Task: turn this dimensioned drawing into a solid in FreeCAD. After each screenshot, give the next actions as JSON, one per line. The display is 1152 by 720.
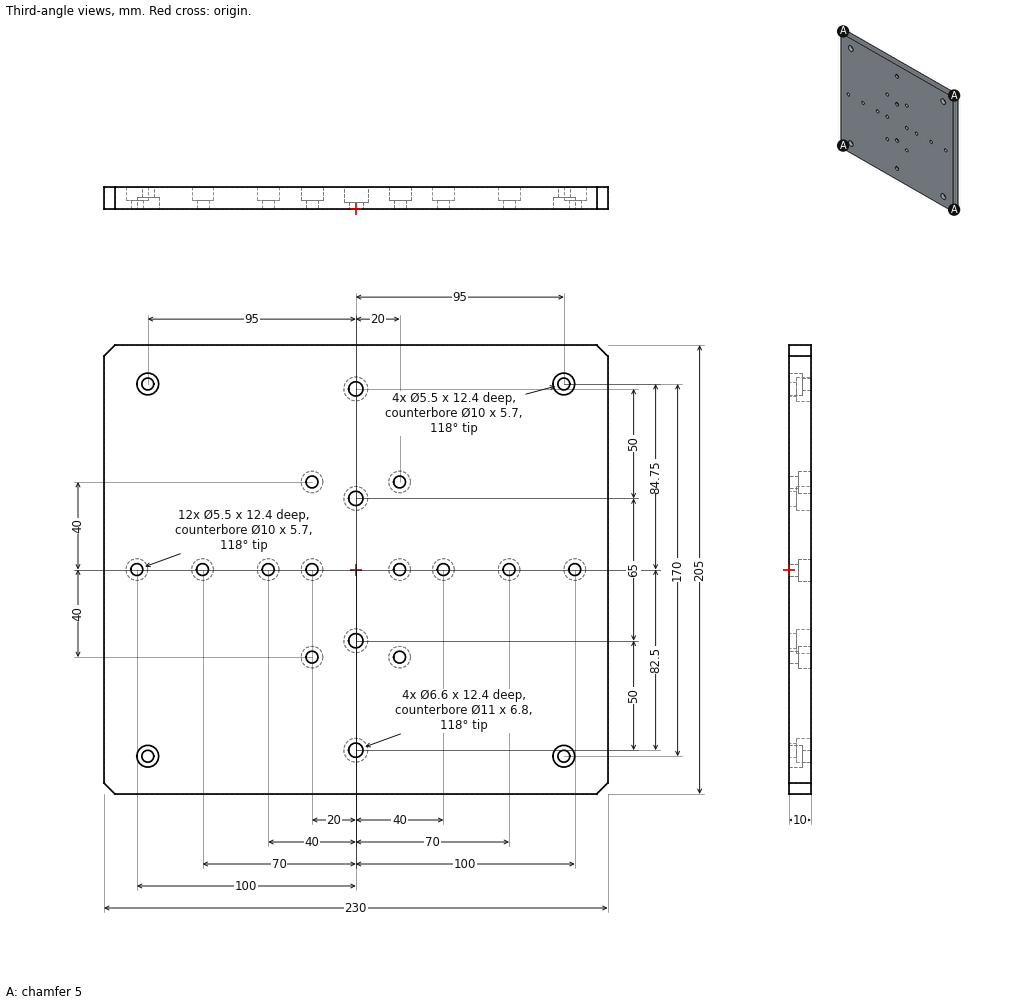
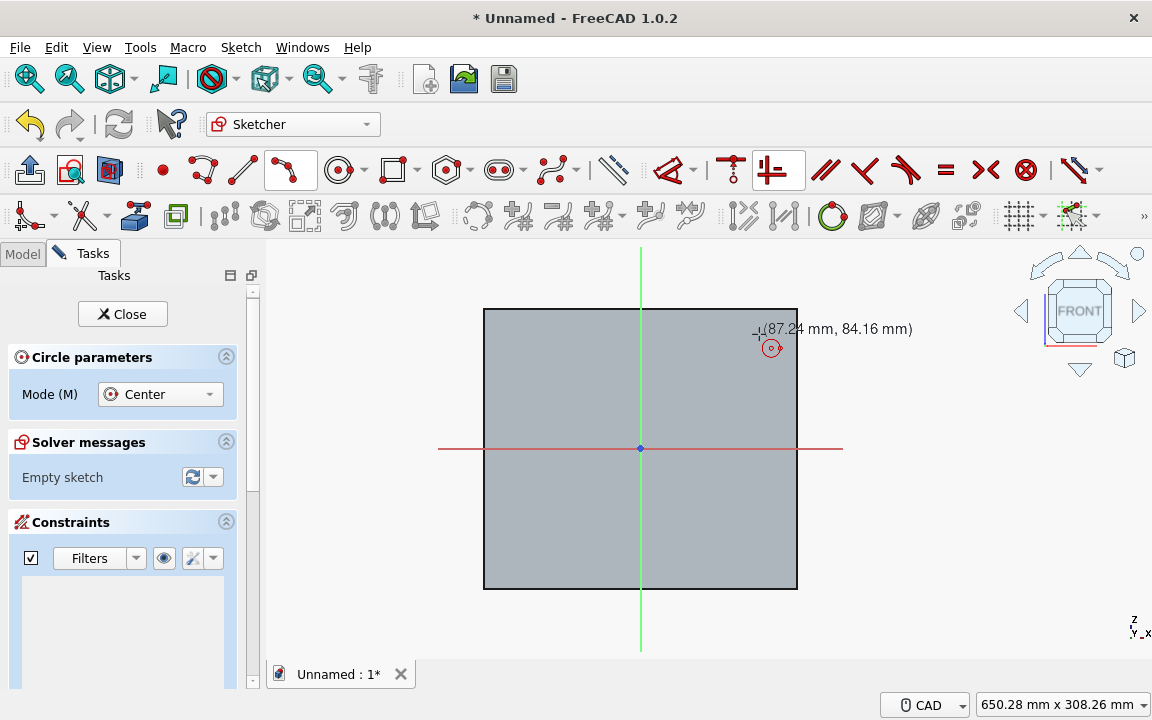
{"action": "left_click", "coordinate": [770, 334]}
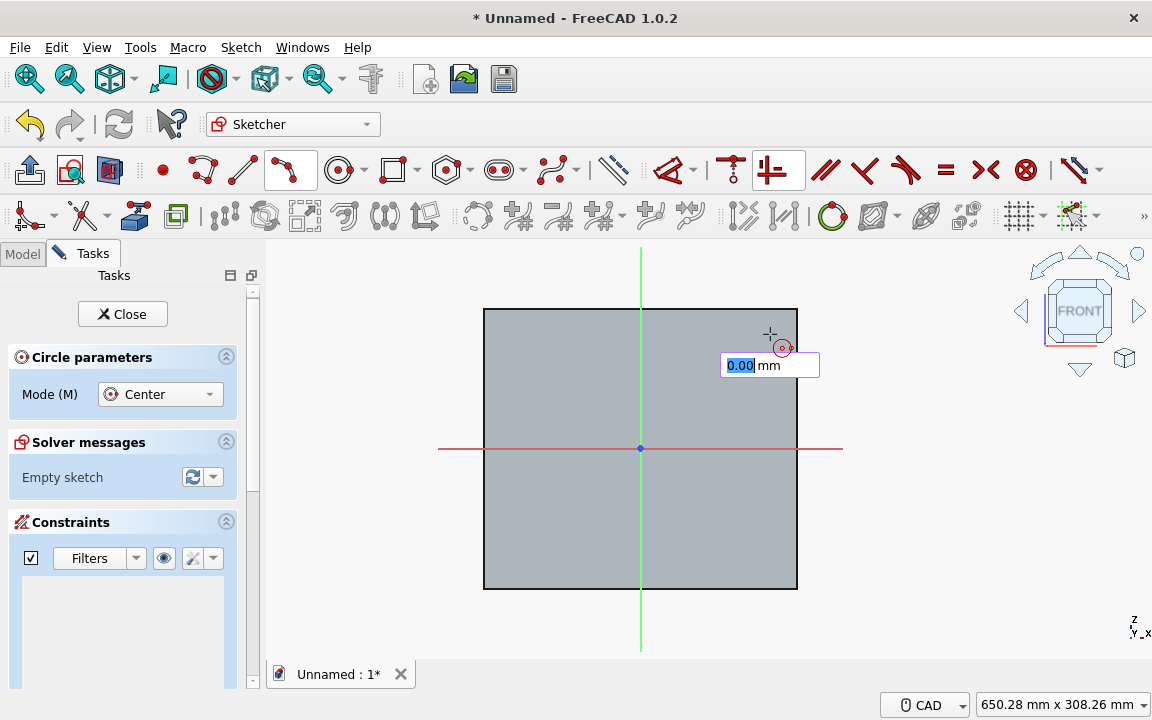
{"action": "scroll", "coordinate": [773, 331], "scroll_direction": "up", "scroll_amount": 8}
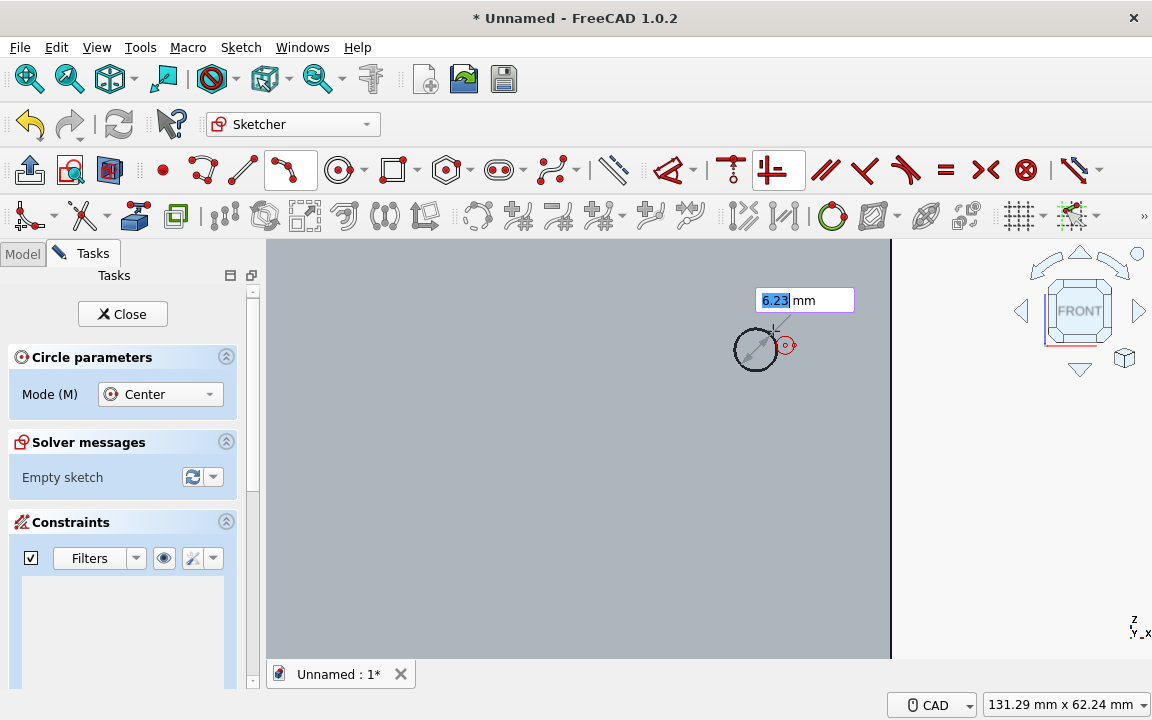
{"action": "left_click", "coordinate": [769, 330]}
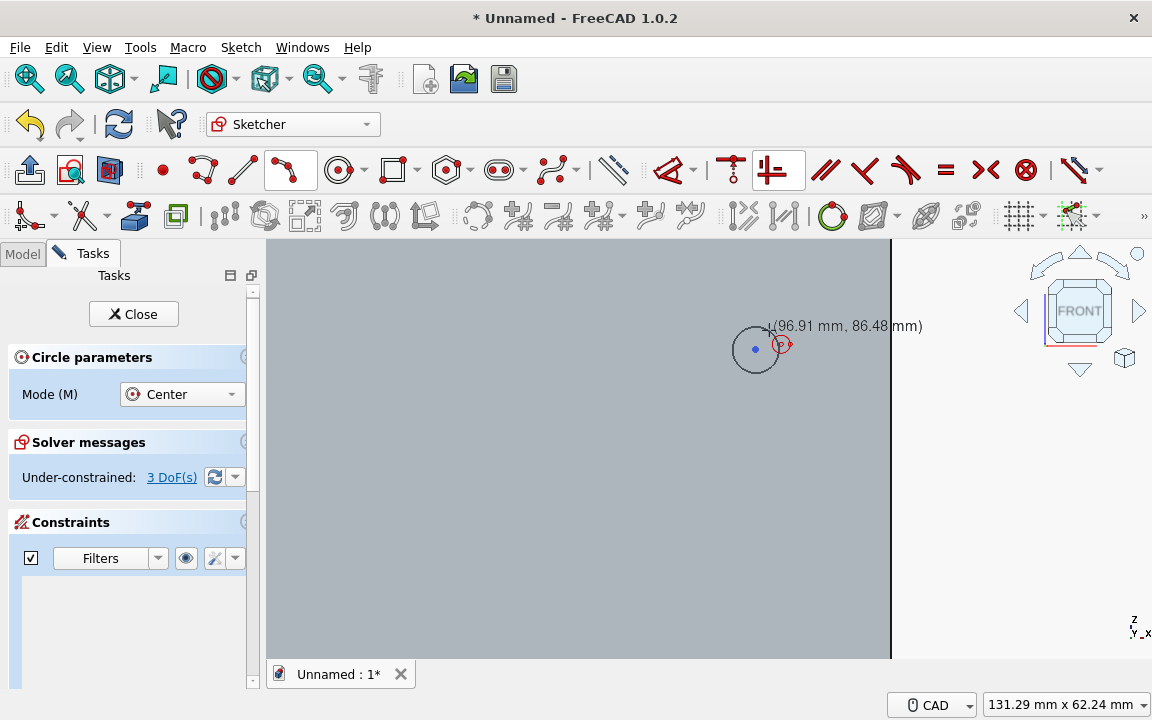
{"action": "scroll", "coordinate": [773, 331], "scroll_direction": "down", "scroll_amount": 8}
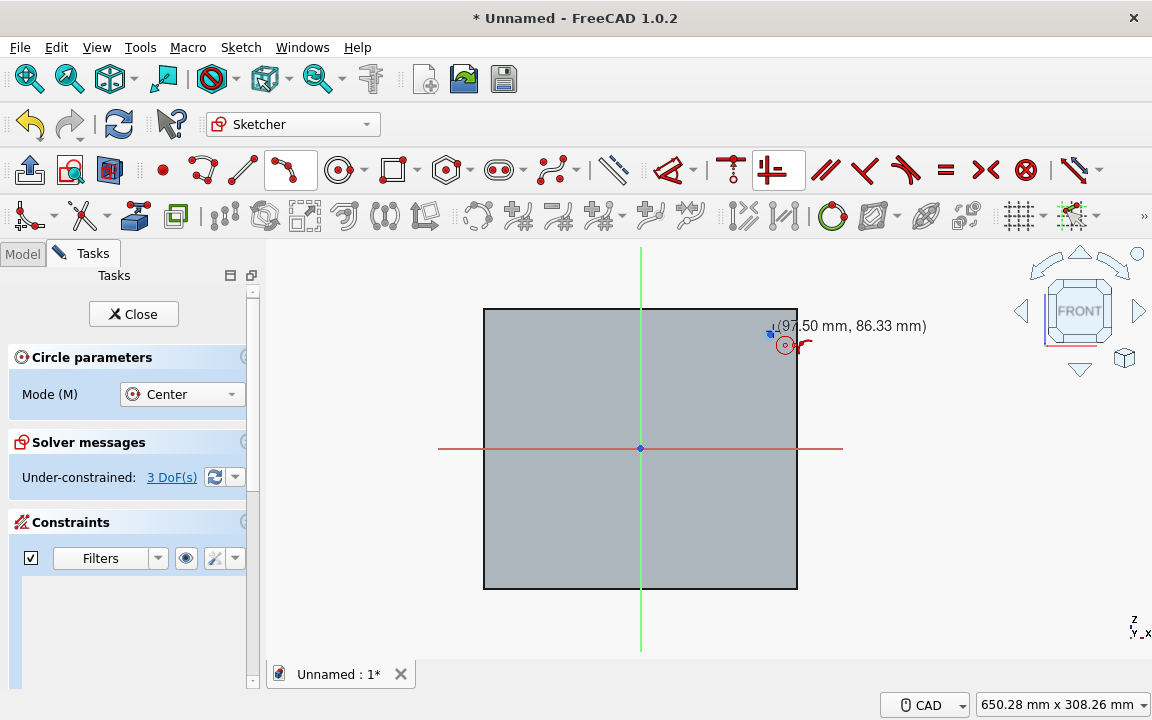
{"action": "scroll", "coordinate": [770, 565], "scroll_direction": "up", "scroll_amount": 10}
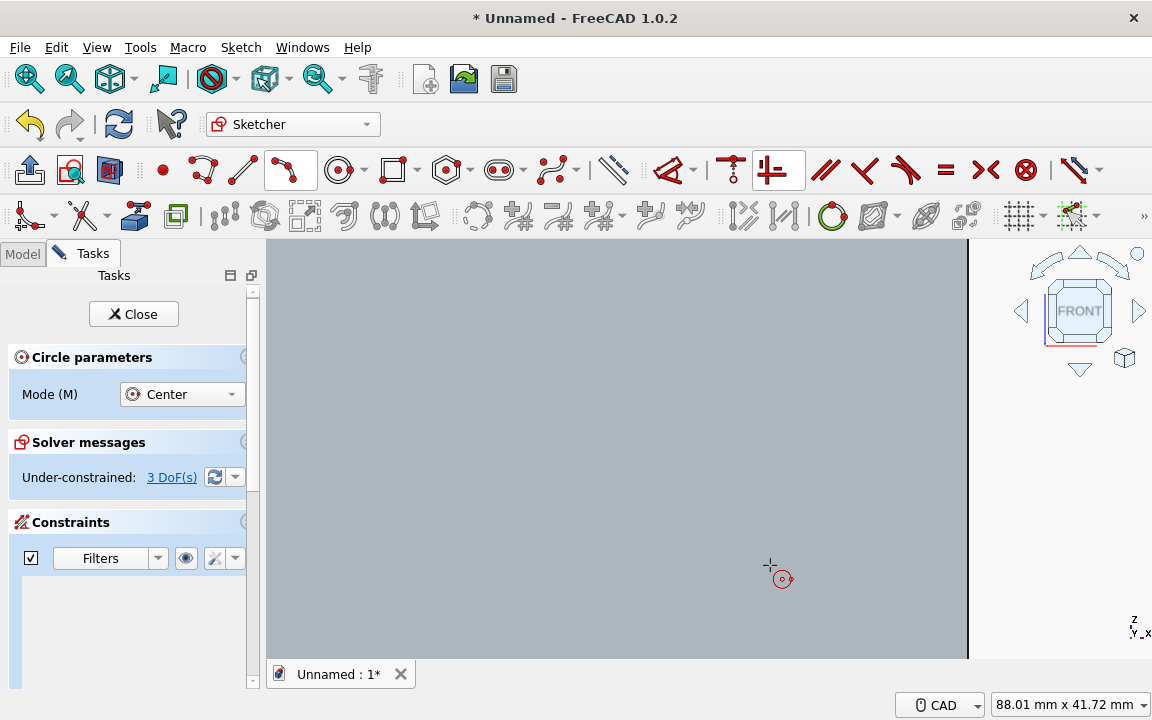
{"action": "scroll", "coordinate": [770, 565], "scroll_direction": "down", "scroll_amount": 10}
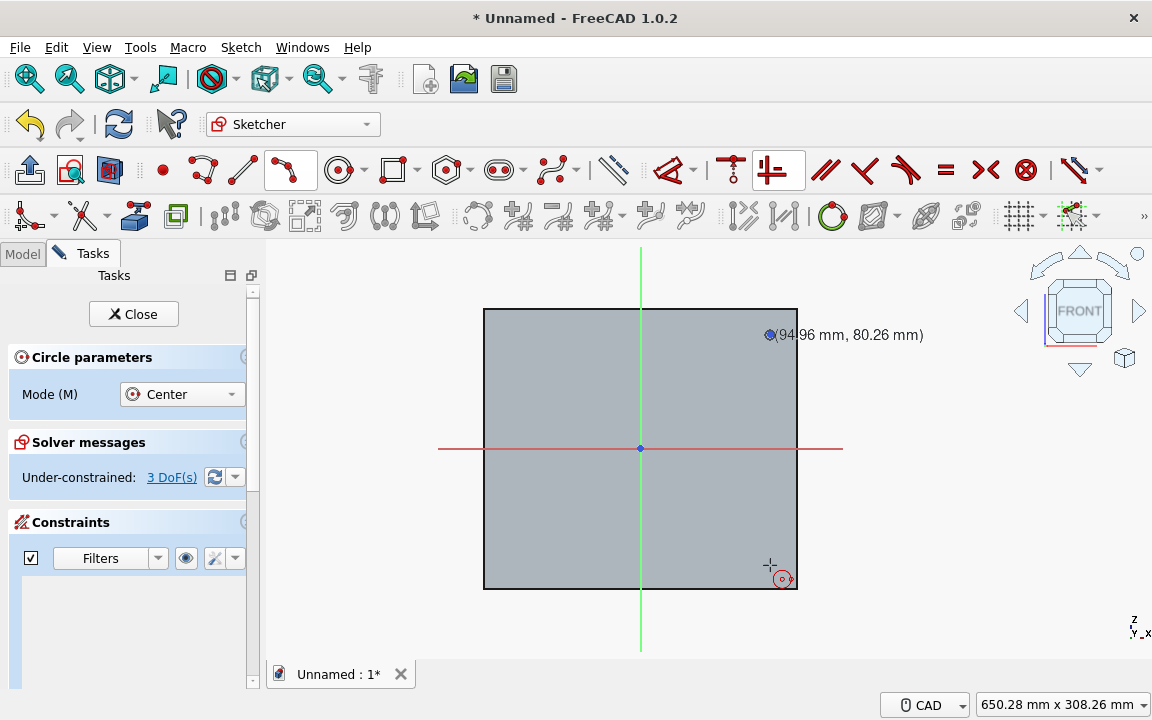
{"action": "left_click", "coordinate": [770, 565]}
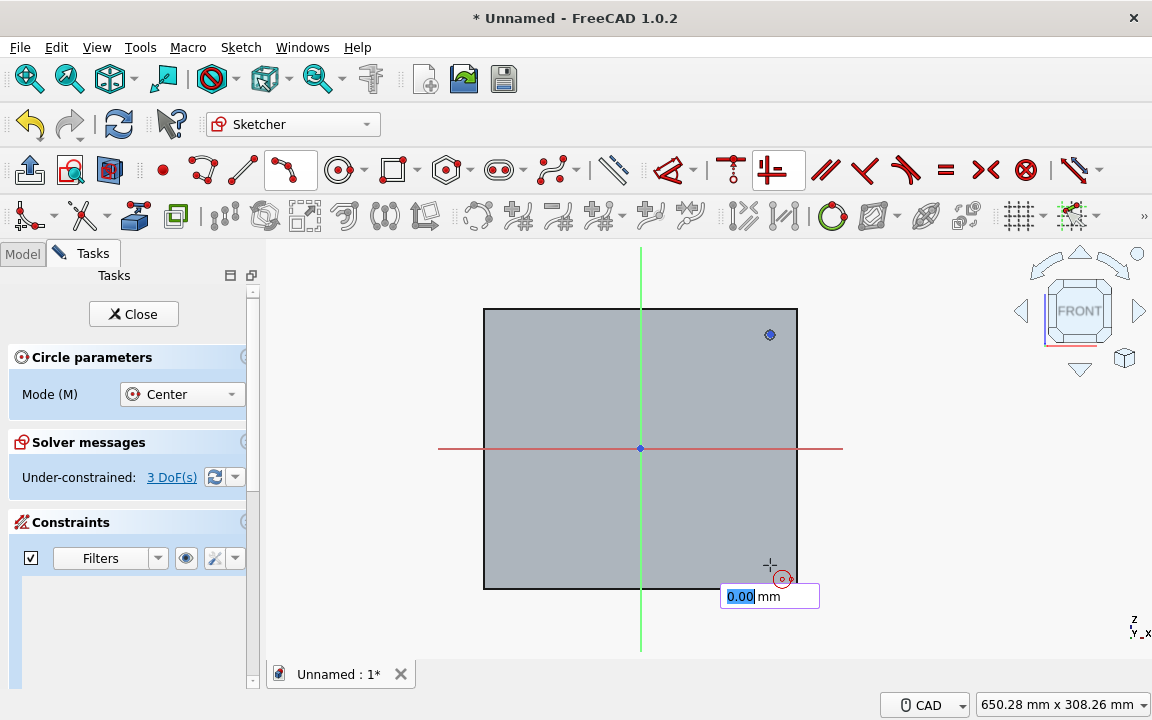
{"action": "scroll", "coordinate": [773, 563], "scroll_direction": "up", "scroll_amount": 8}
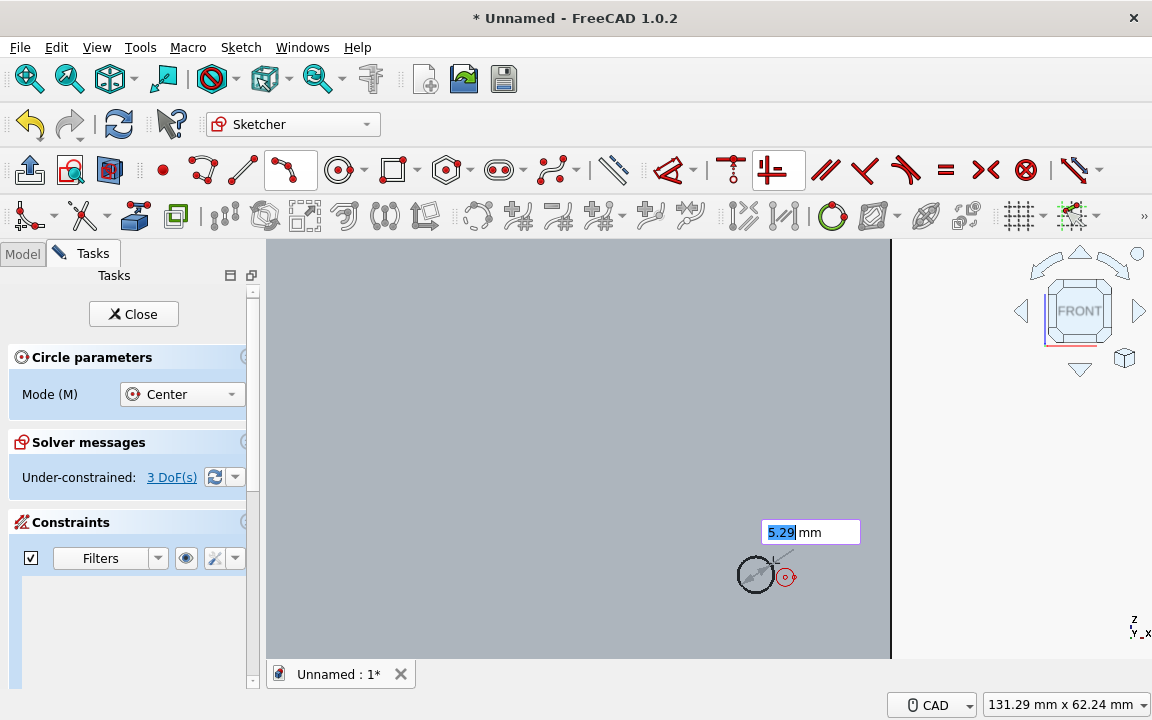
{"action": "left_click", "coordinate": [769, 557]}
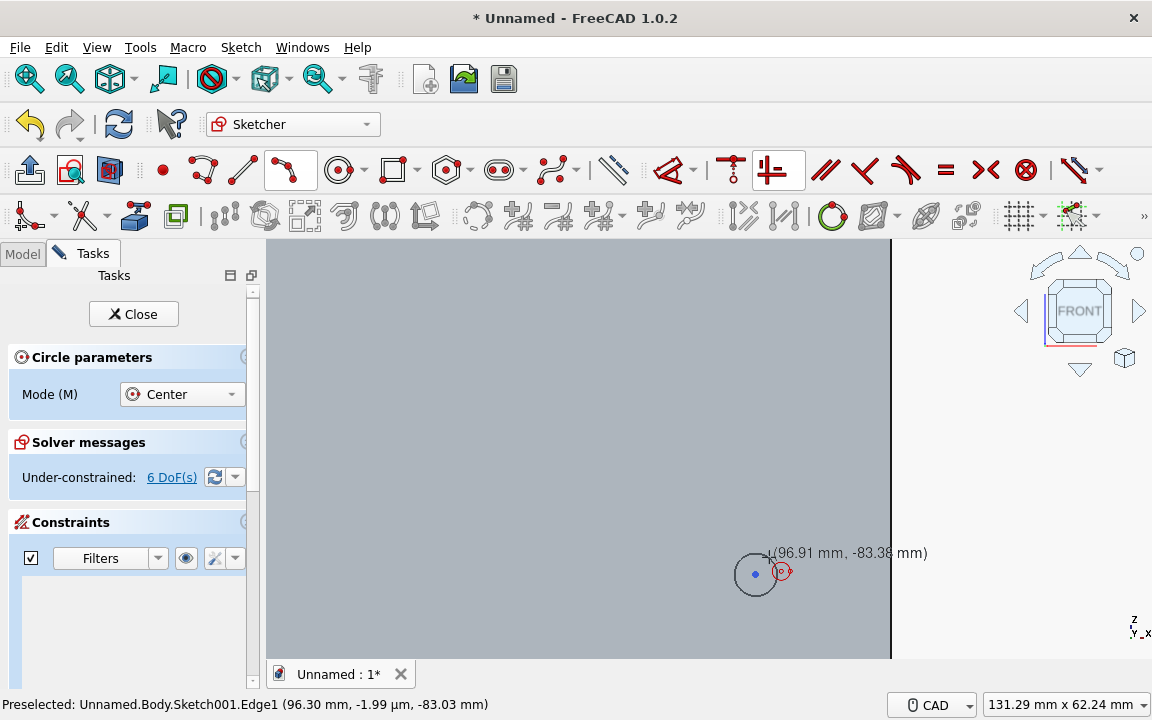
{"action": "scroll", "coordinate": [773, 563], "scroll_direction": "down", "scroll_amount": 8}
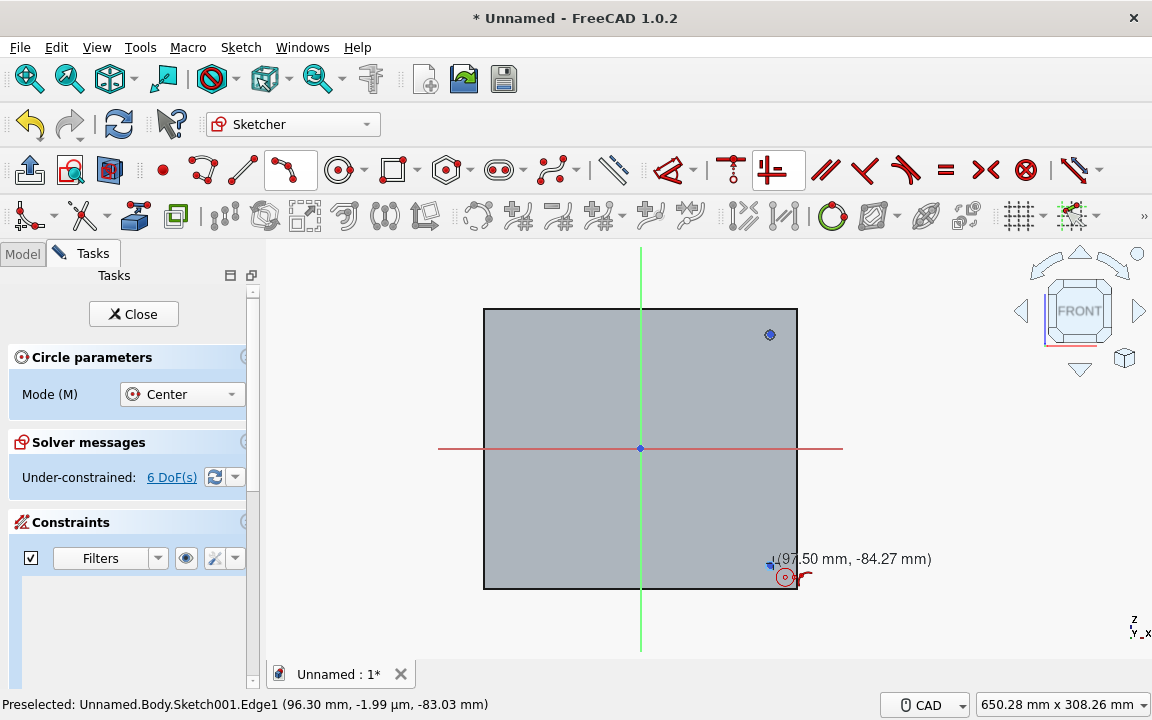
{"action": "scroll", "coordinate": [511, 334], "scroll_direction": "up", "scroll_amount": 10}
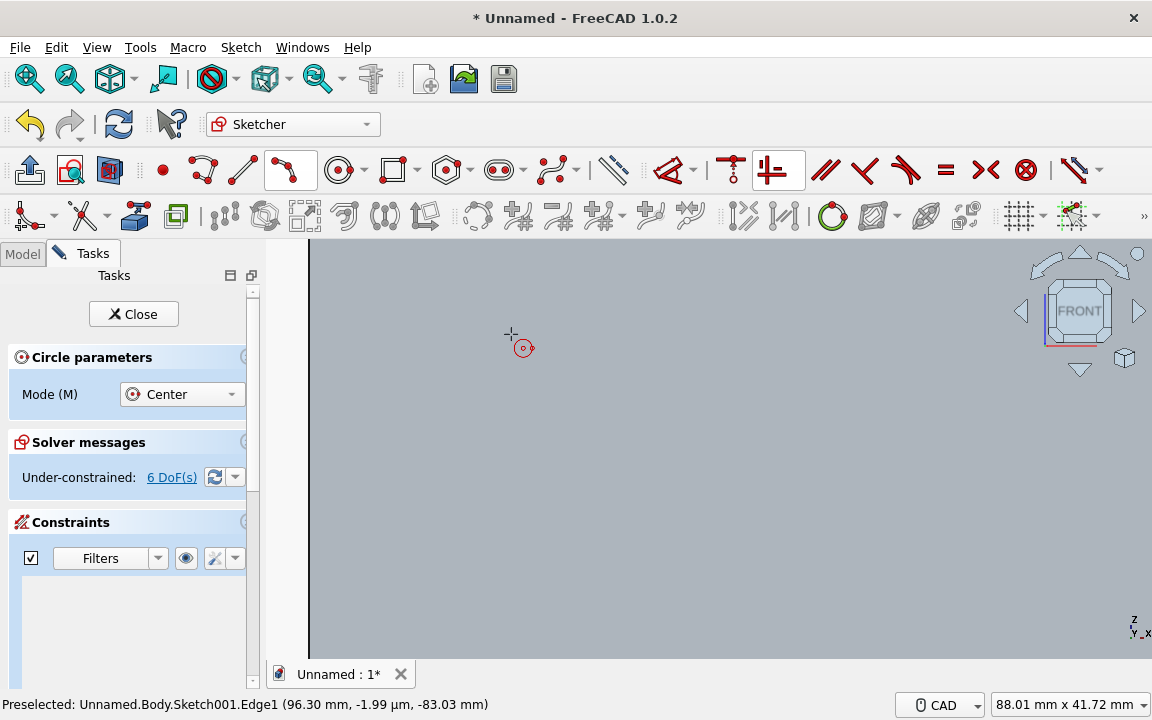
{"action": "scroll", "coordinate": [511, 334], "scroll_direction": "down", "scroll_amount": 10}